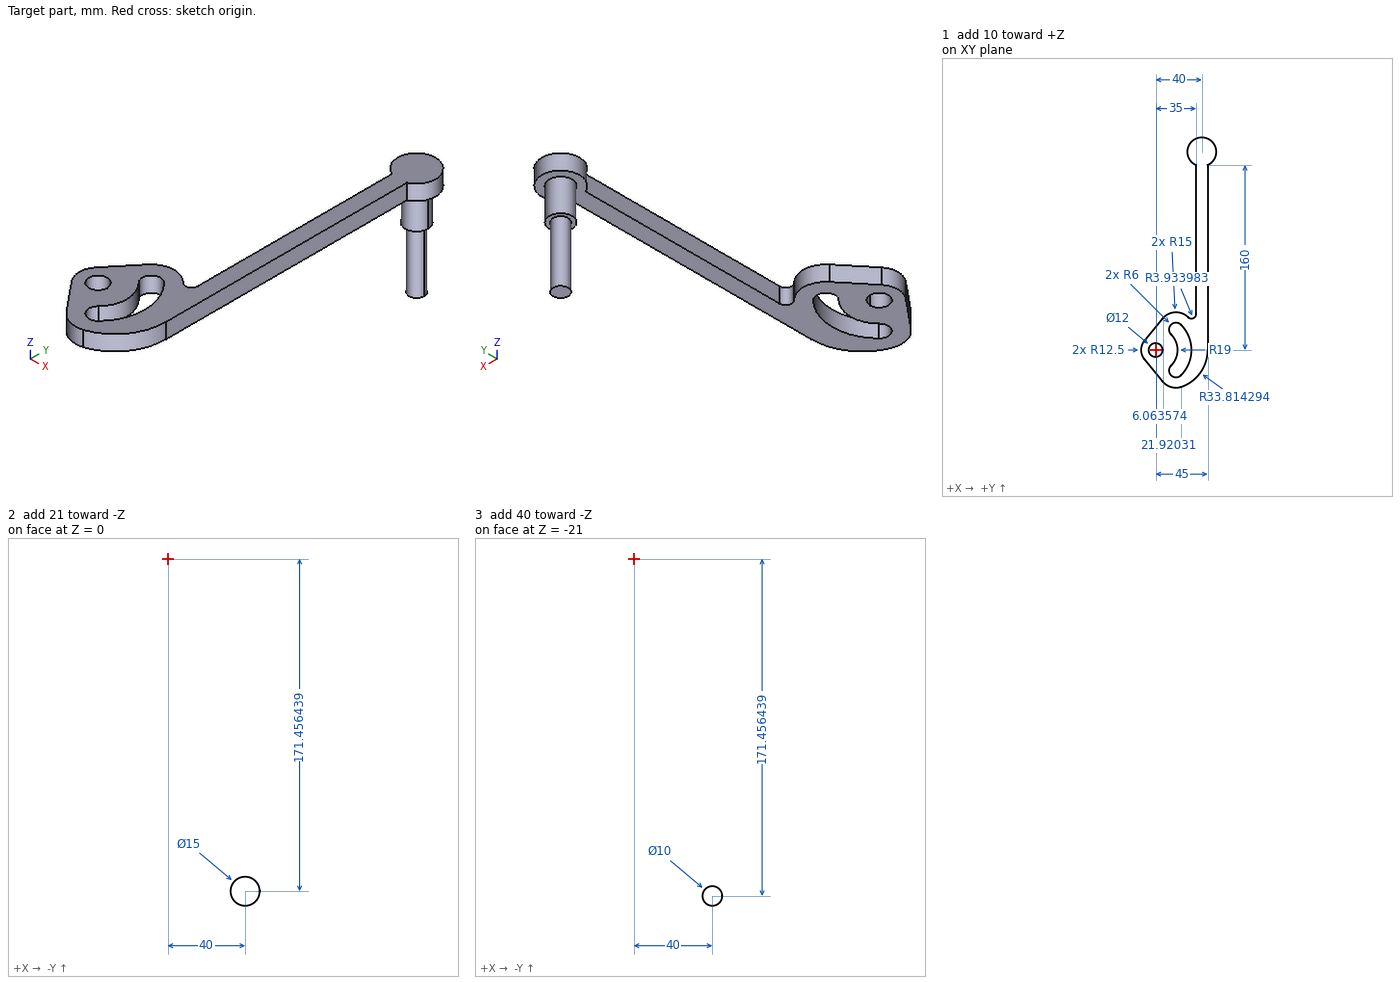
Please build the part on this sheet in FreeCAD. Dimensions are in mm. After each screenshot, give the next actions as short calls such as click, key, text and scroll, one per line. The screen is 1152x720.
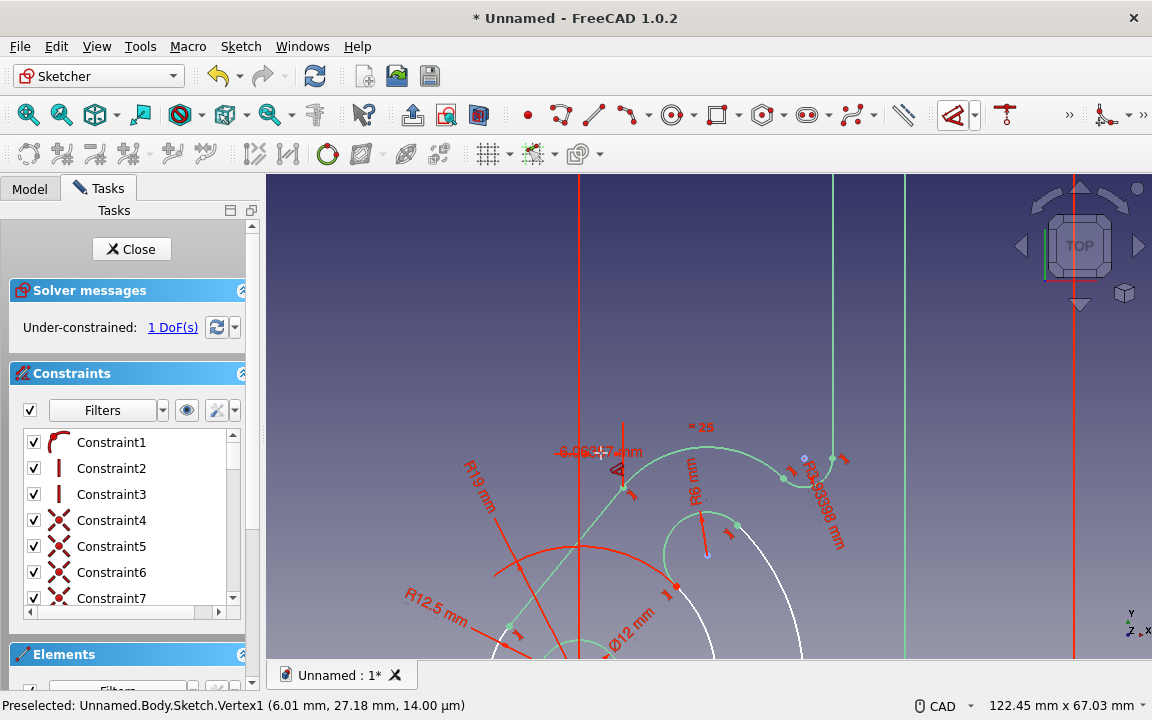
scroll(626, 488, down, 8)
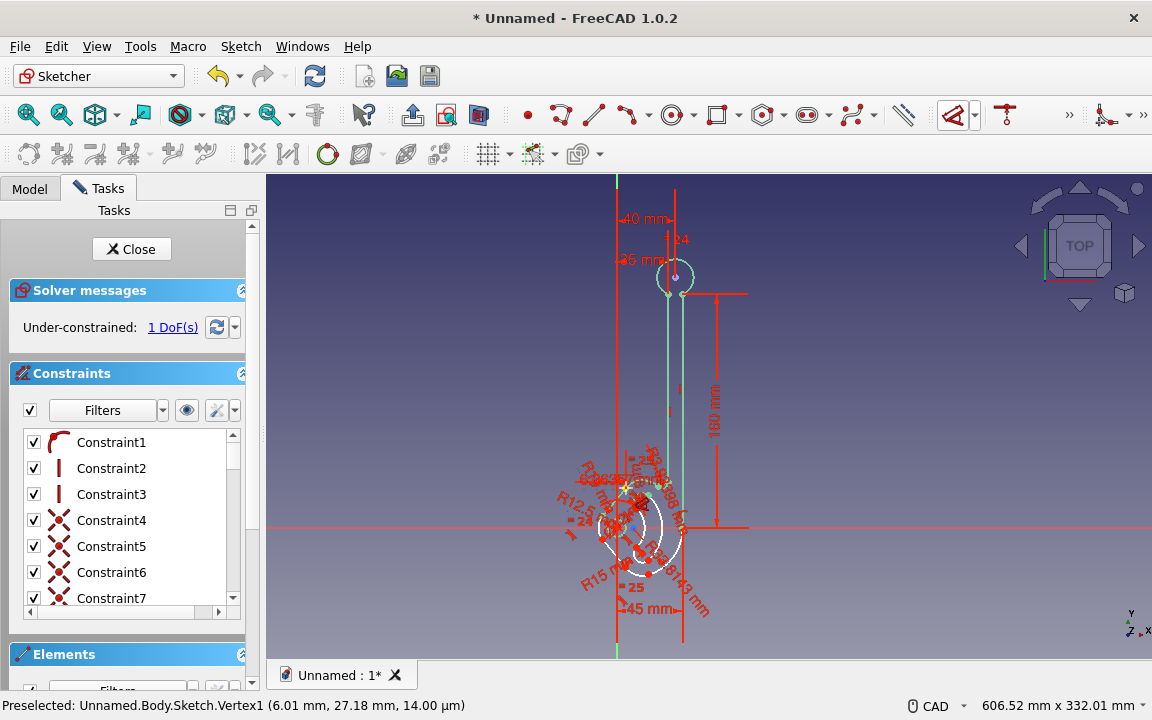
scroll(649, 575, up, 2)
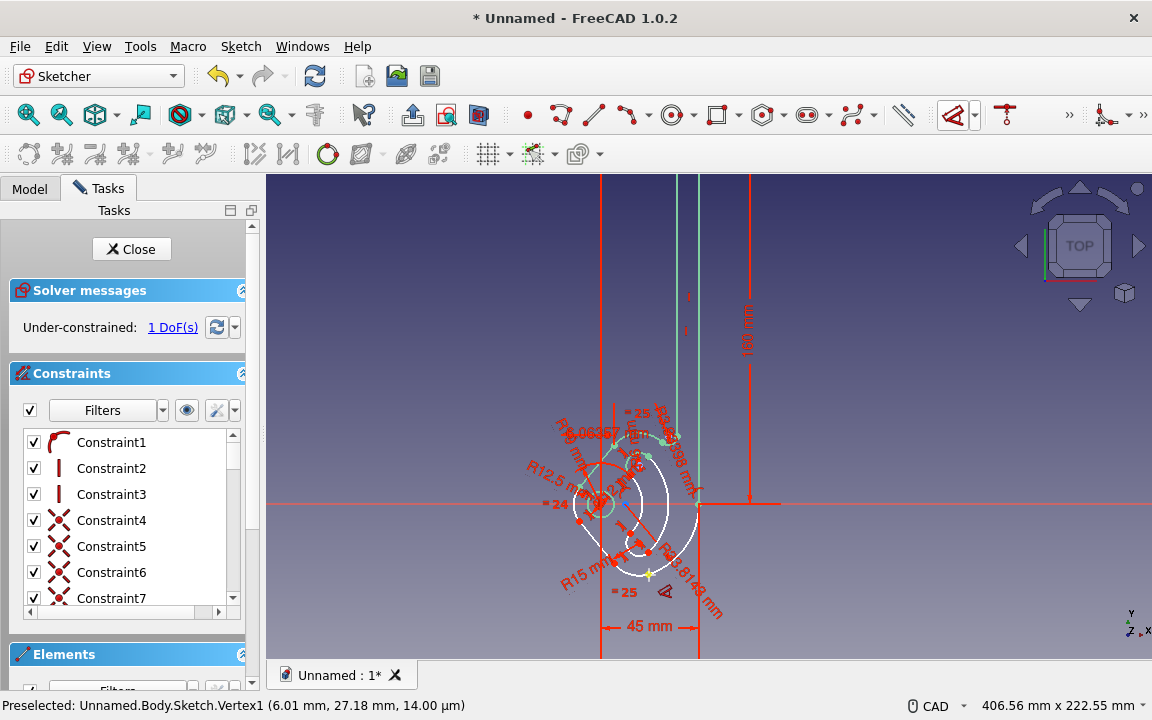
click(648, 574)
click(625, 398)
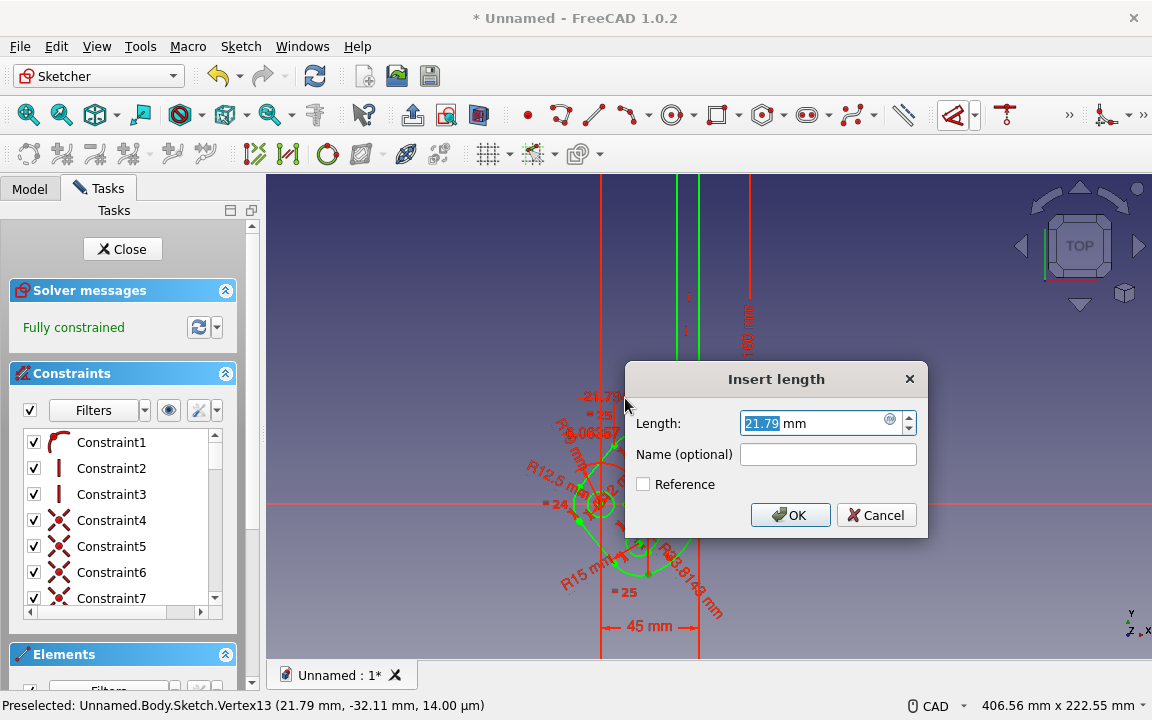
text(21.92031)
key(Return)
key(Escape)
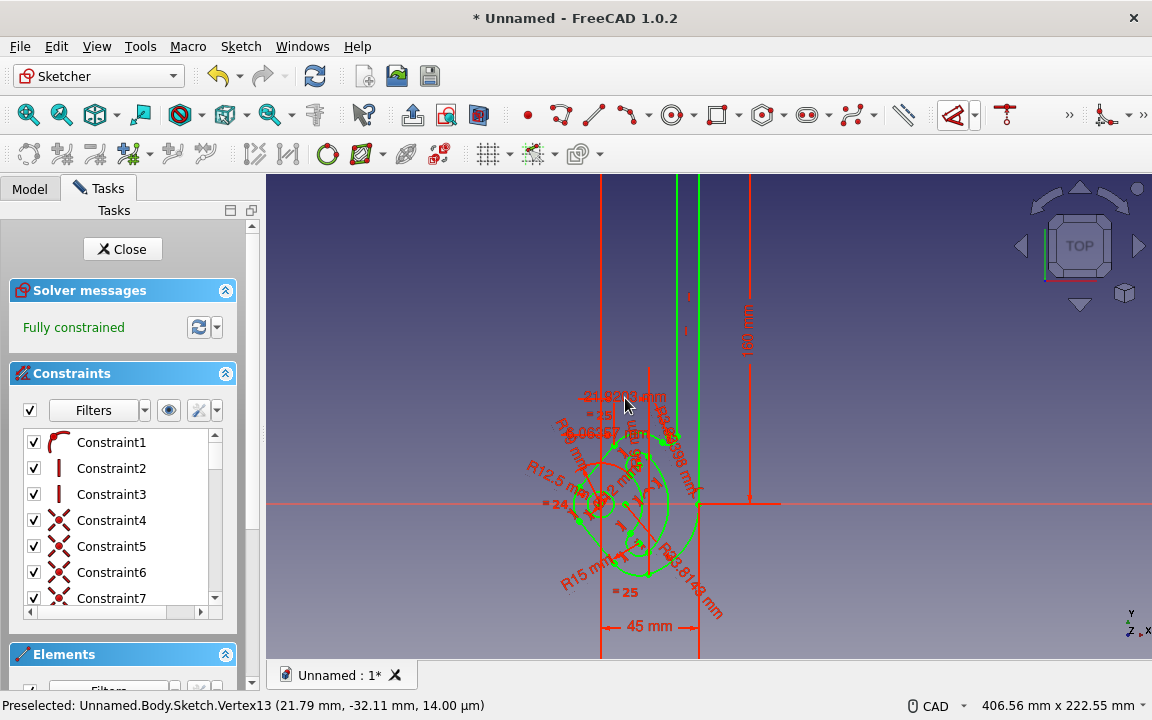
click(123, 249)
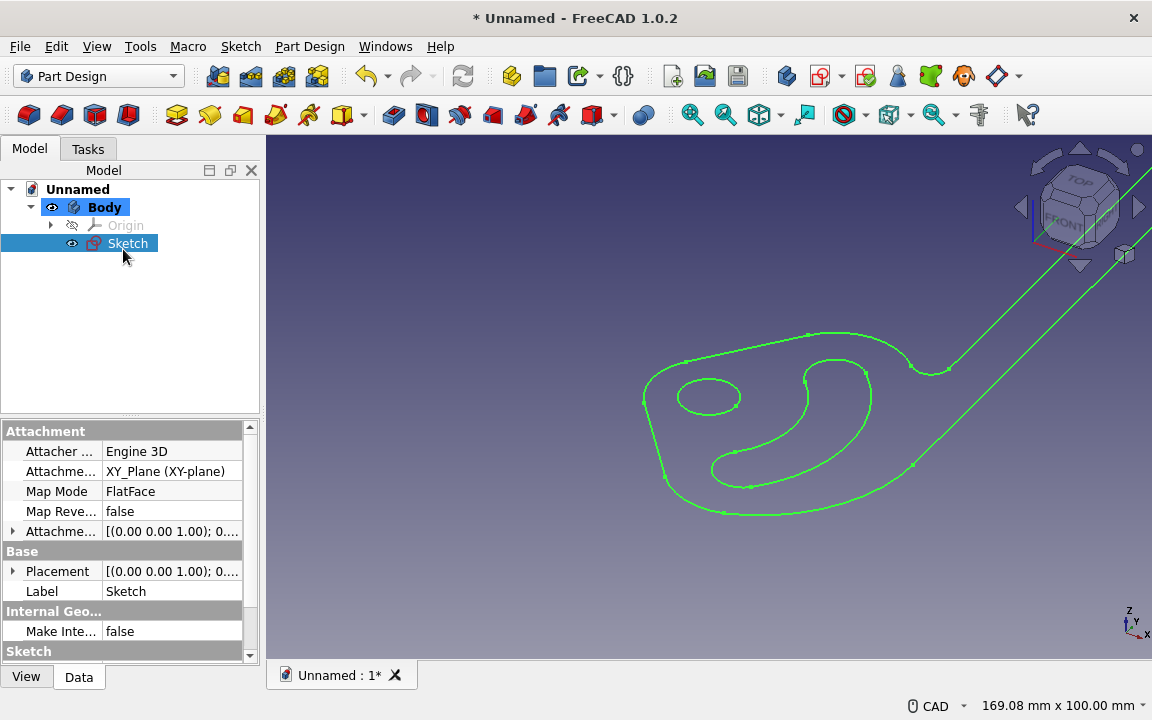
click(177, 116)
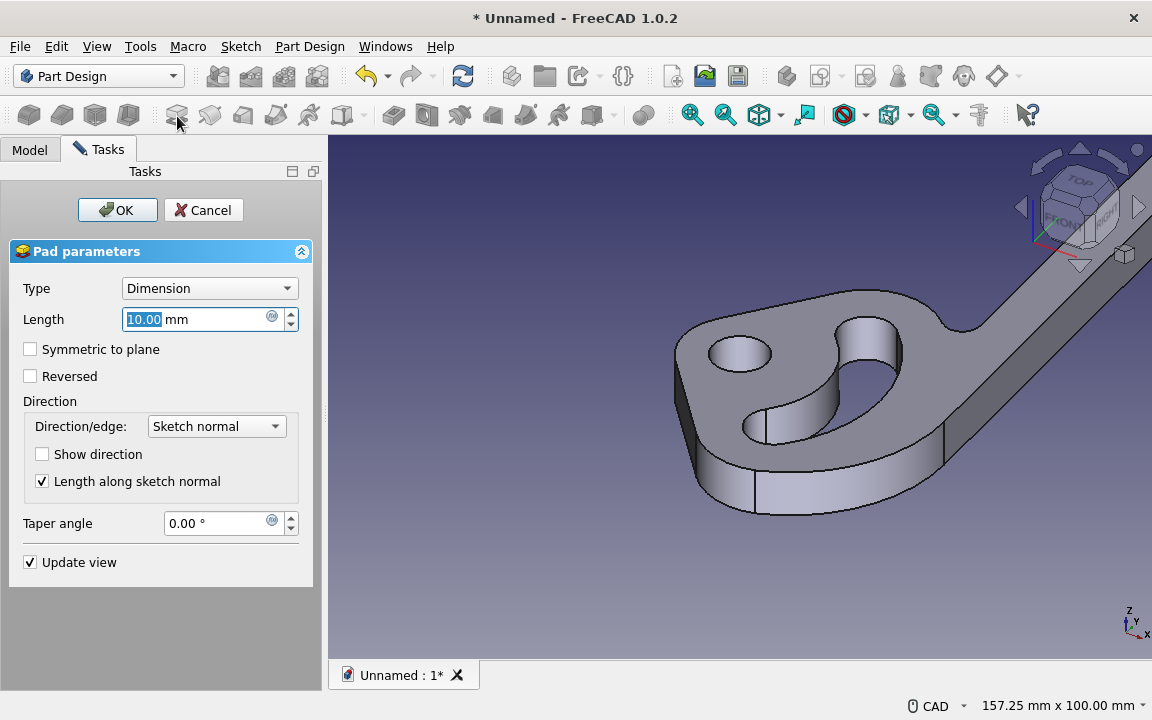
text(10)
key(Tab)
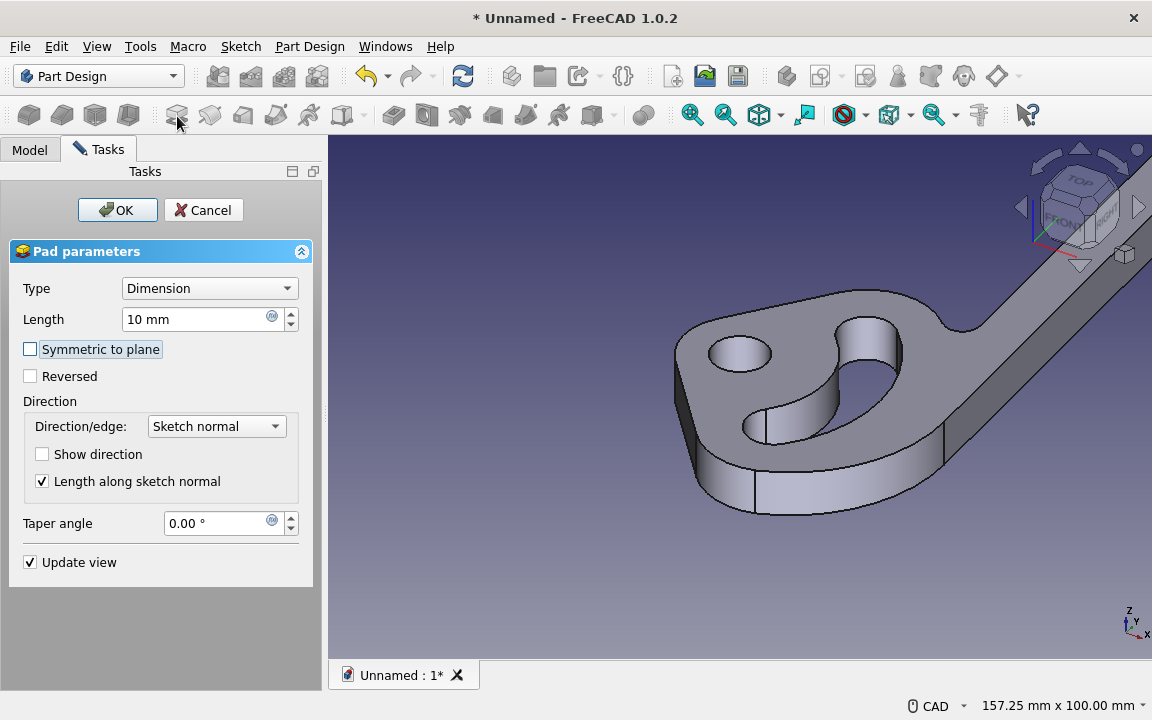
click(118, 210)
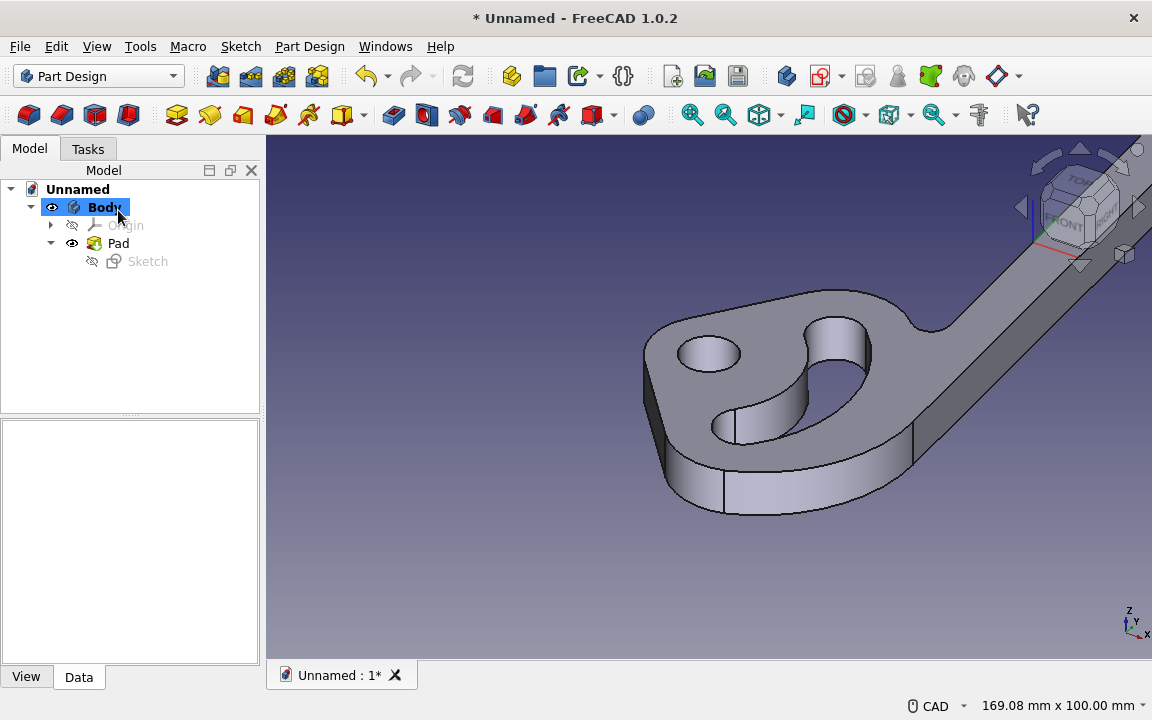
key(v)
key(f)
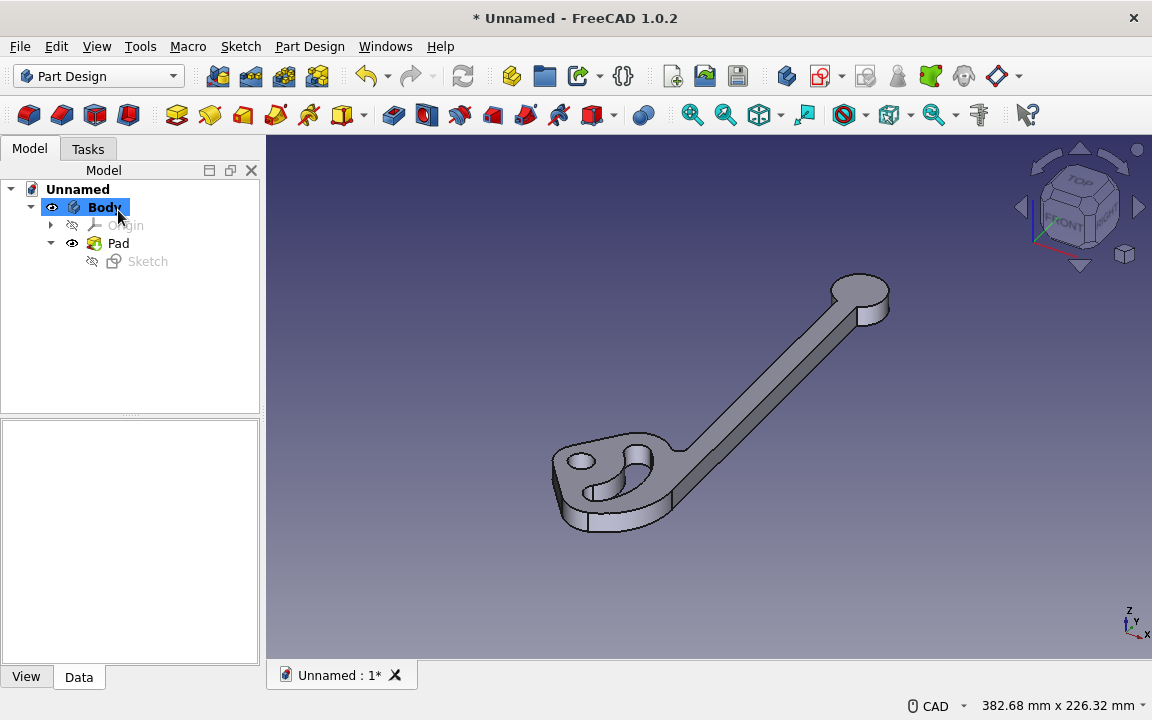
key(5)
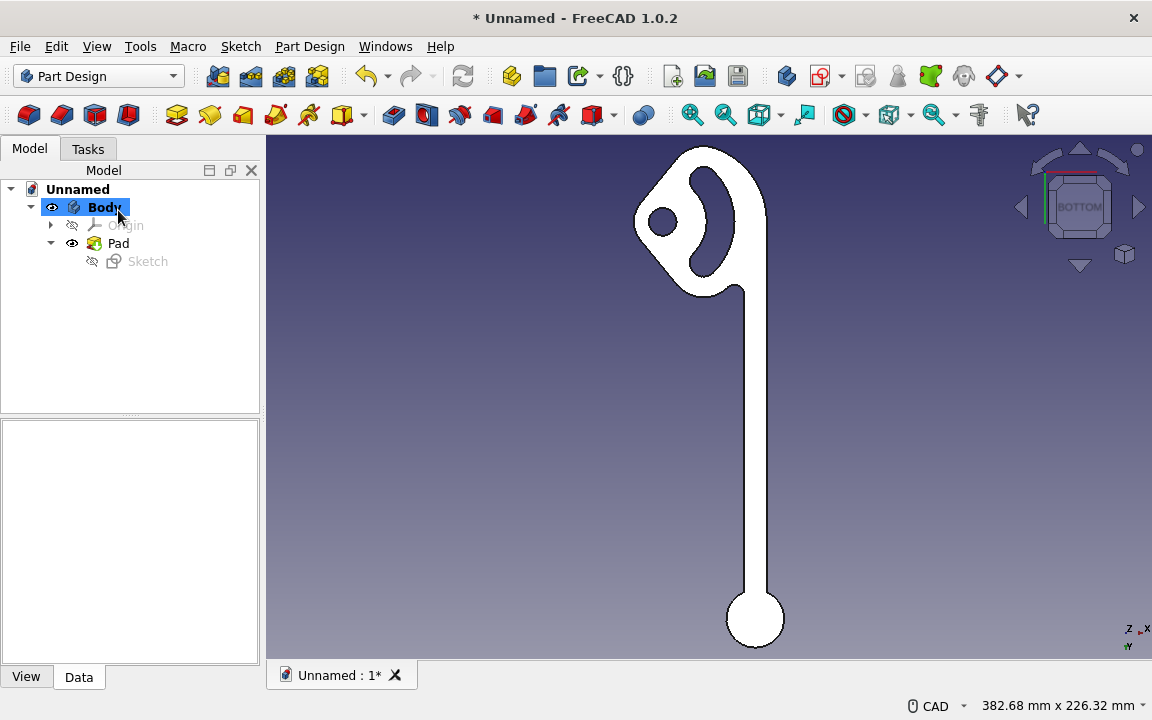
click(752, 611)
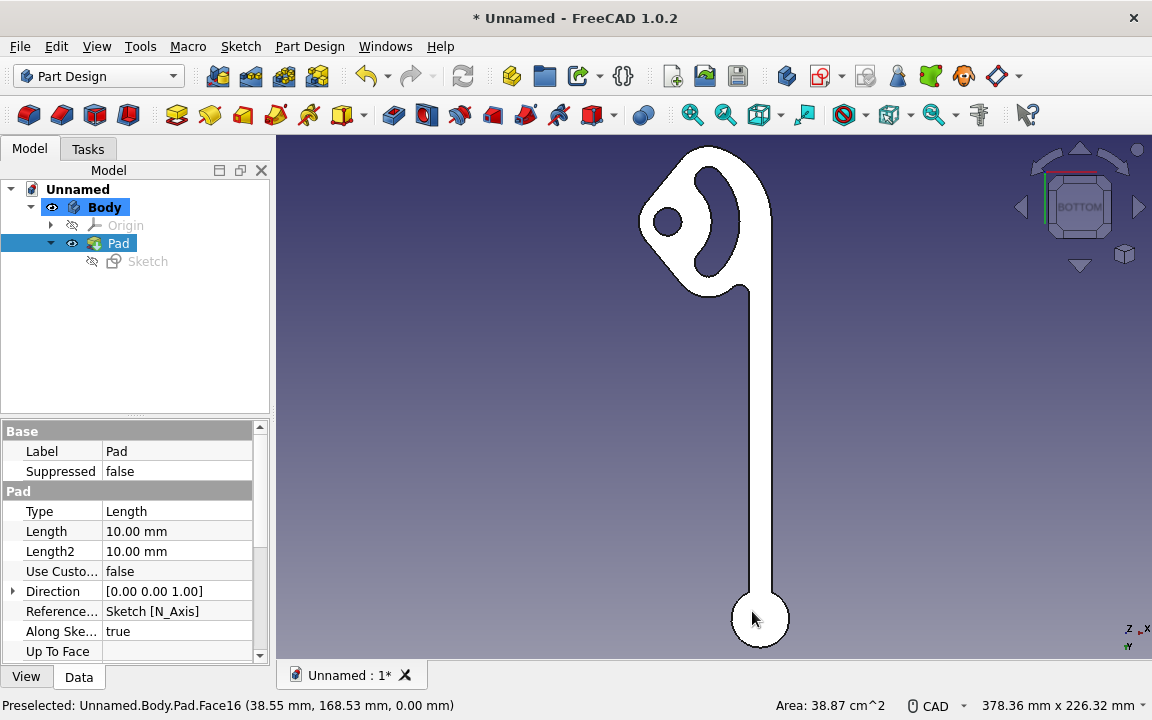
click(820, 76)